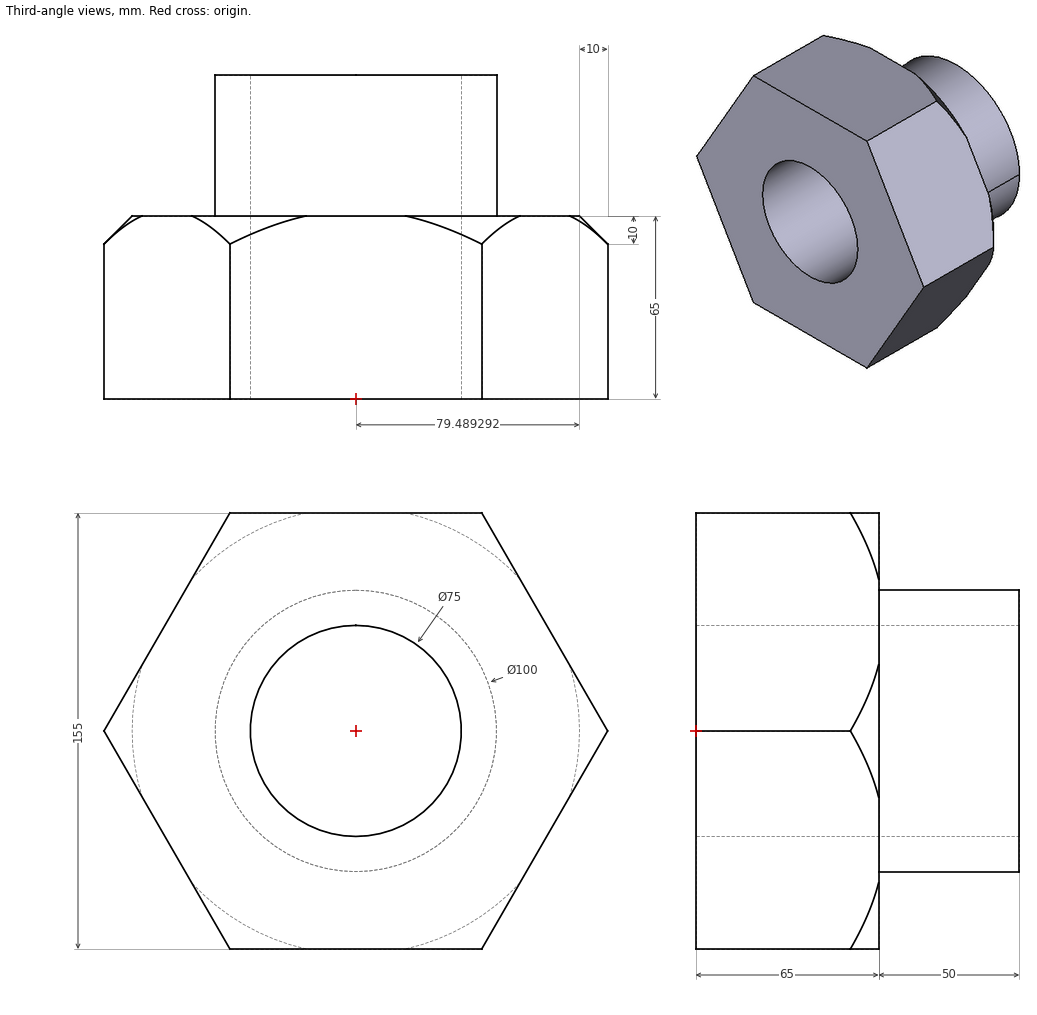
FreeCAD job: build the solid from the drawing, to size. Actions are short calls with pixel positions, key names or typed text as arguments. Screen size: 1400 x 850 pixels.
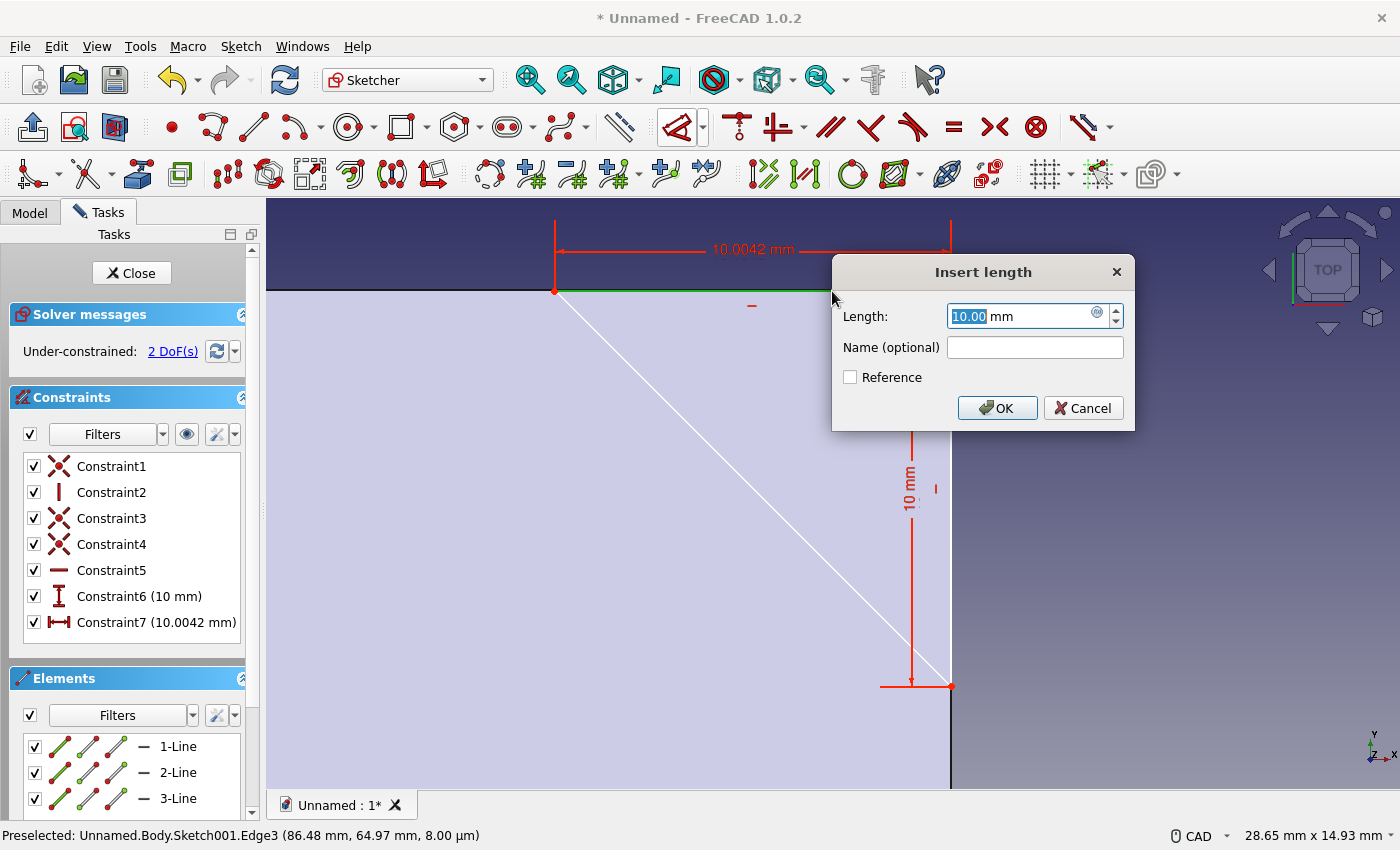
text(10)
key(Return)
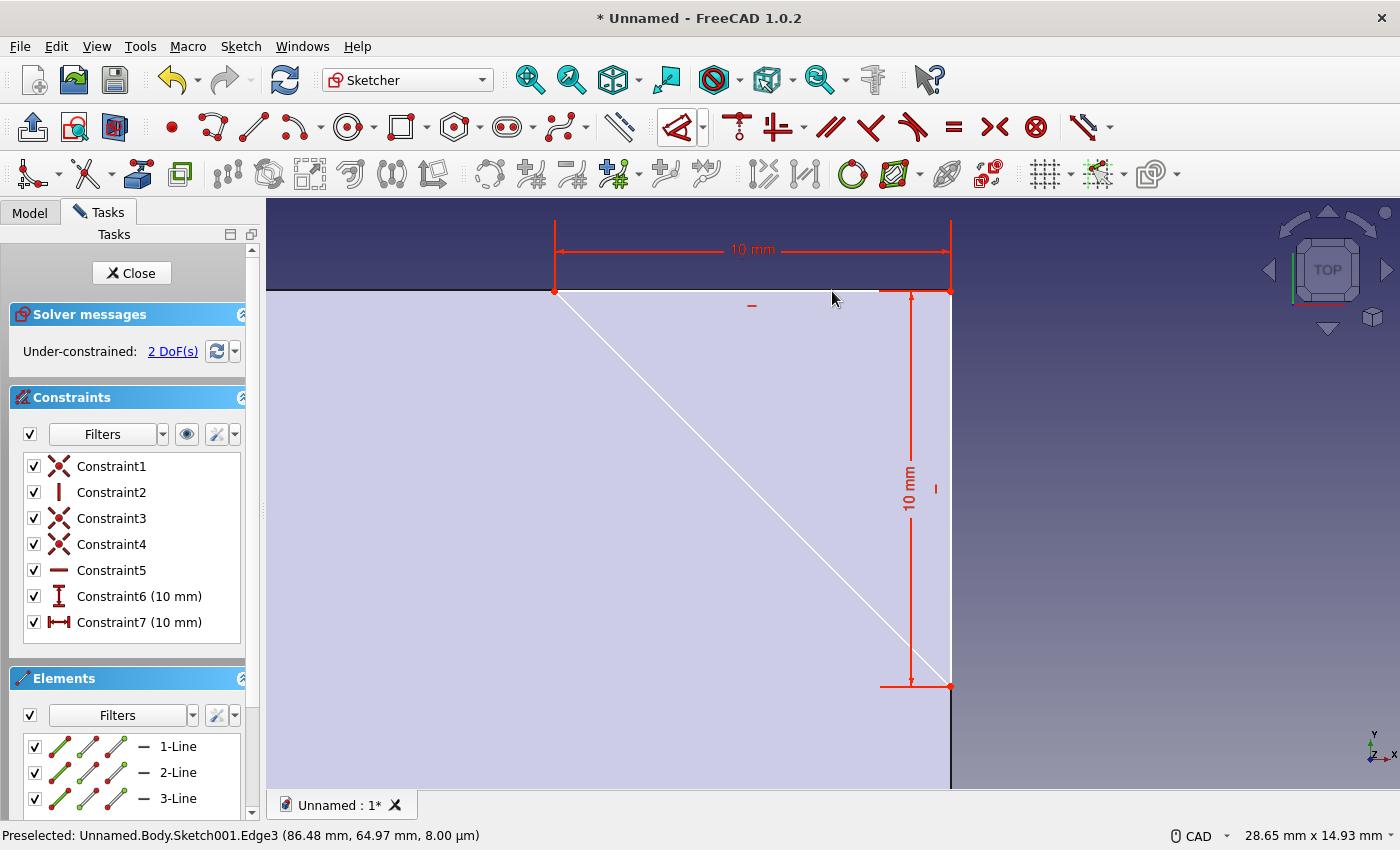
click(555, 291)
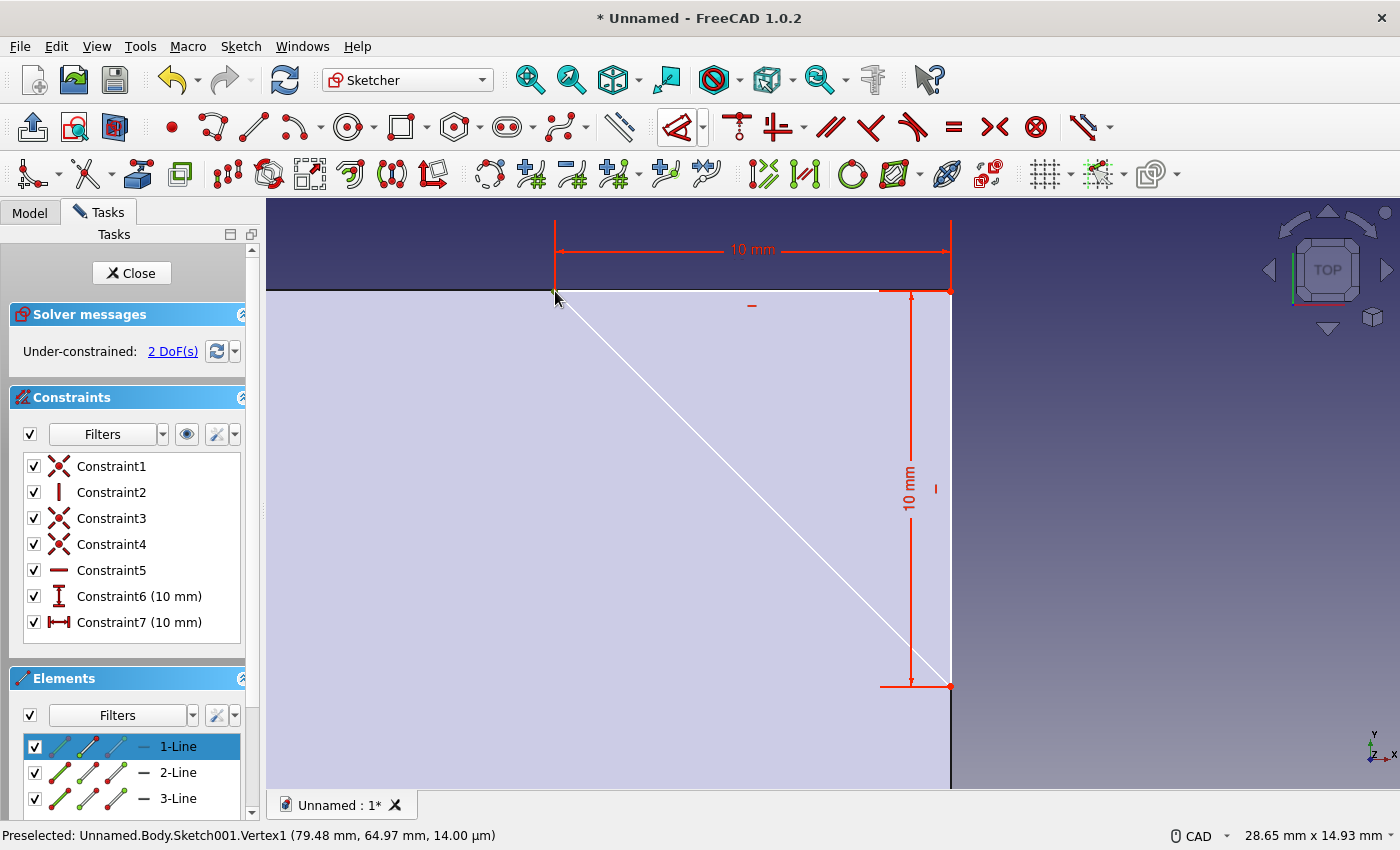
key(i)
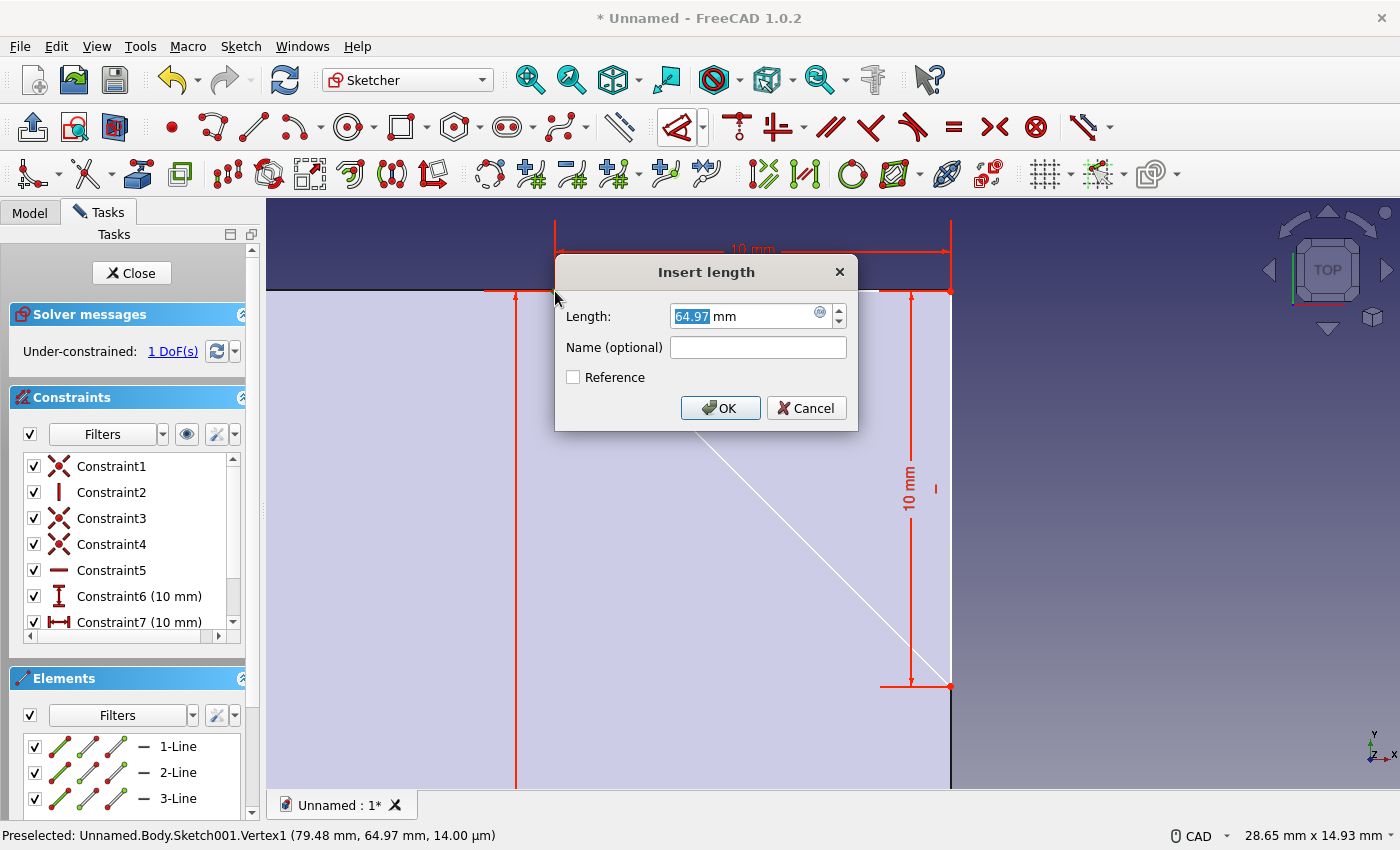
text(65)
key(Return)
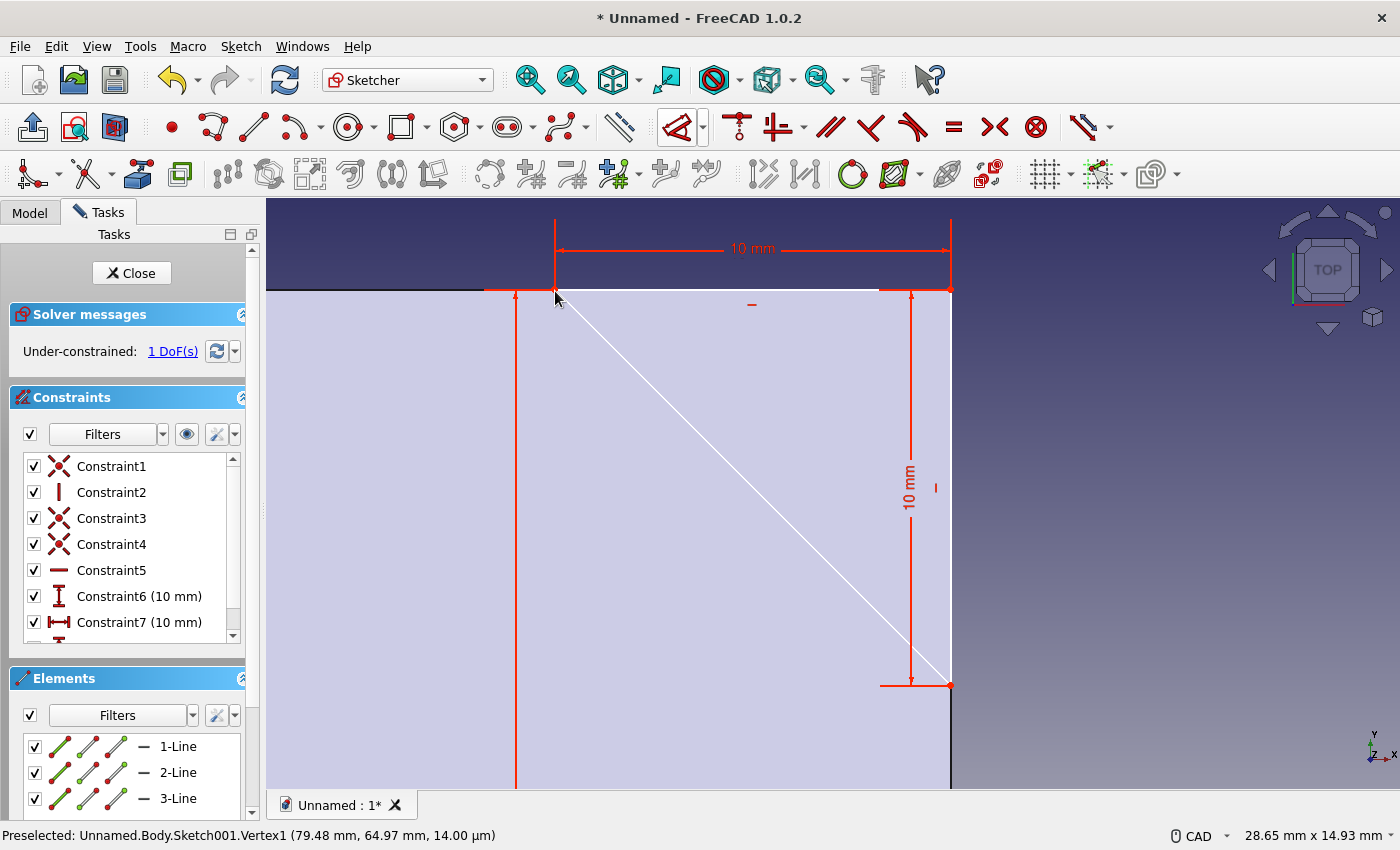
click(555, 290)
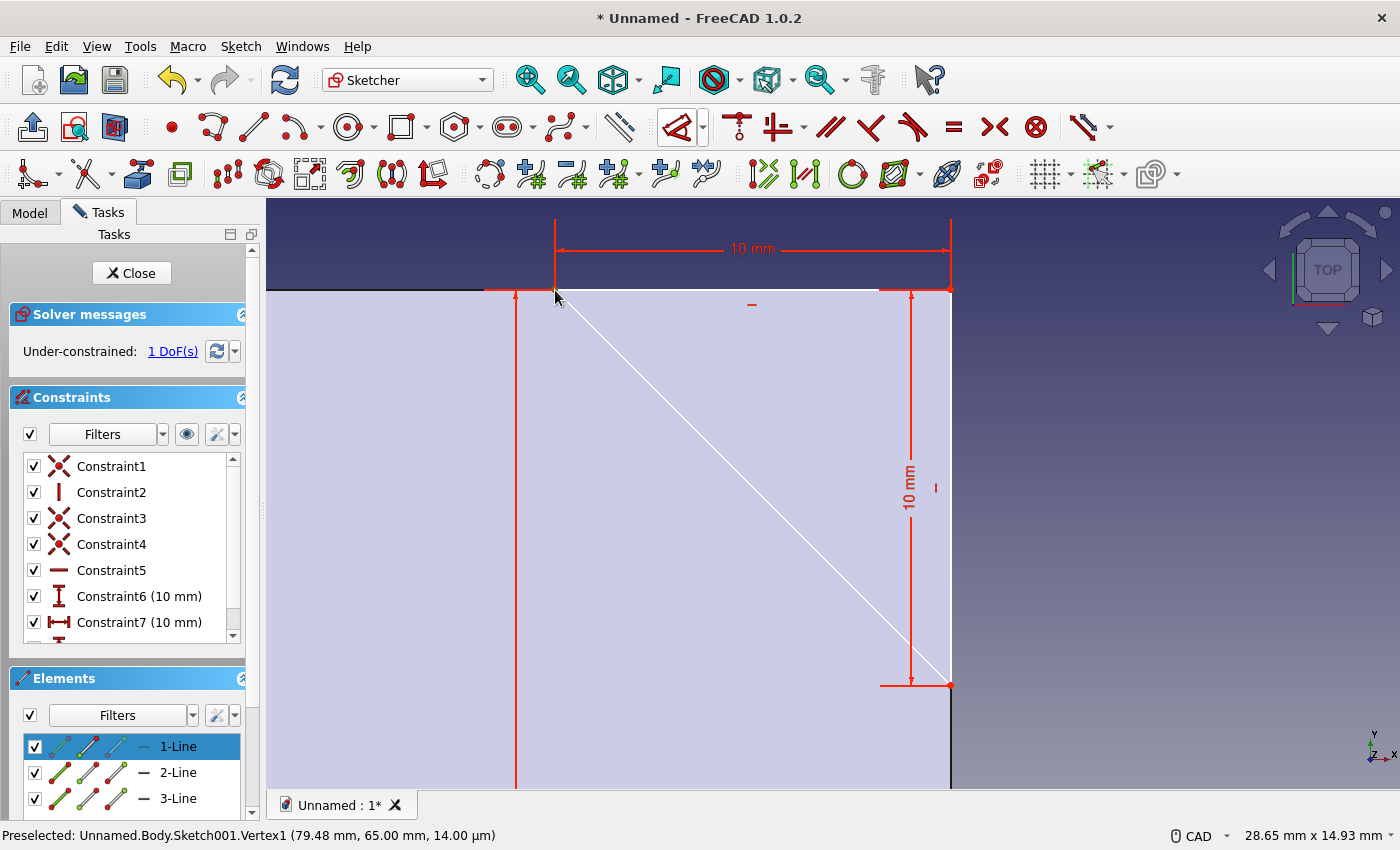
click(702, 128)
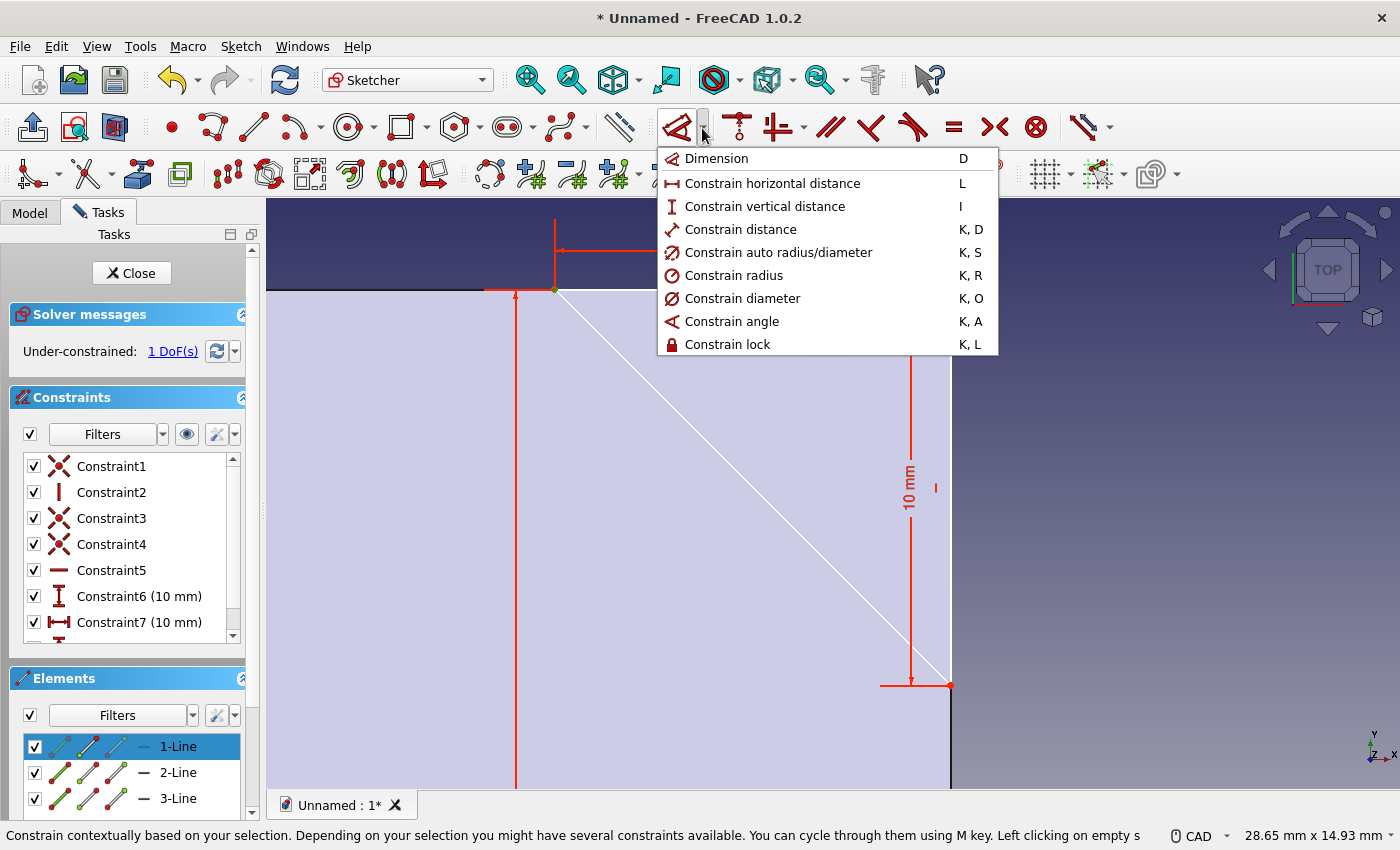
click(828, 184)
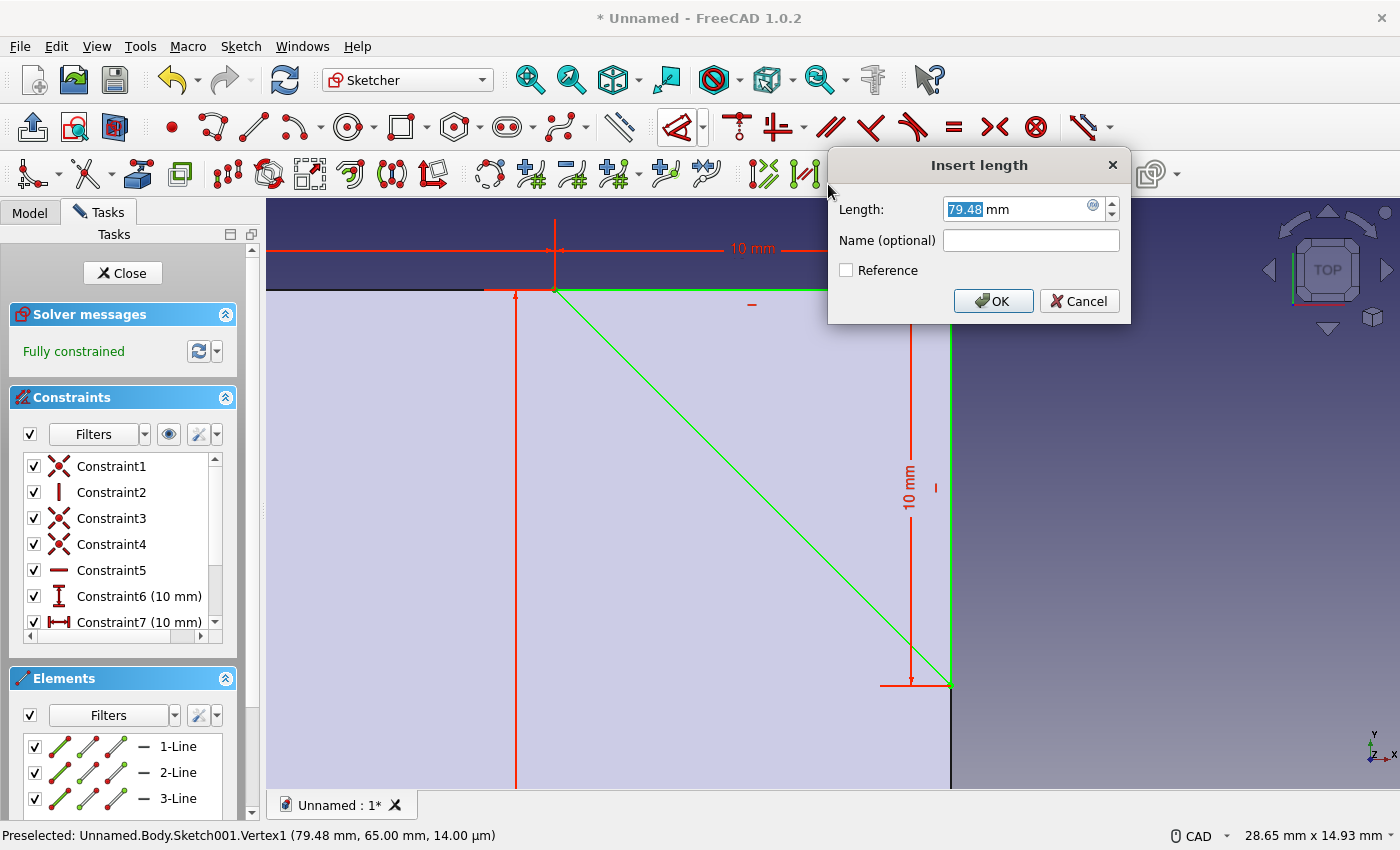
text(79.489292)
key(Return)